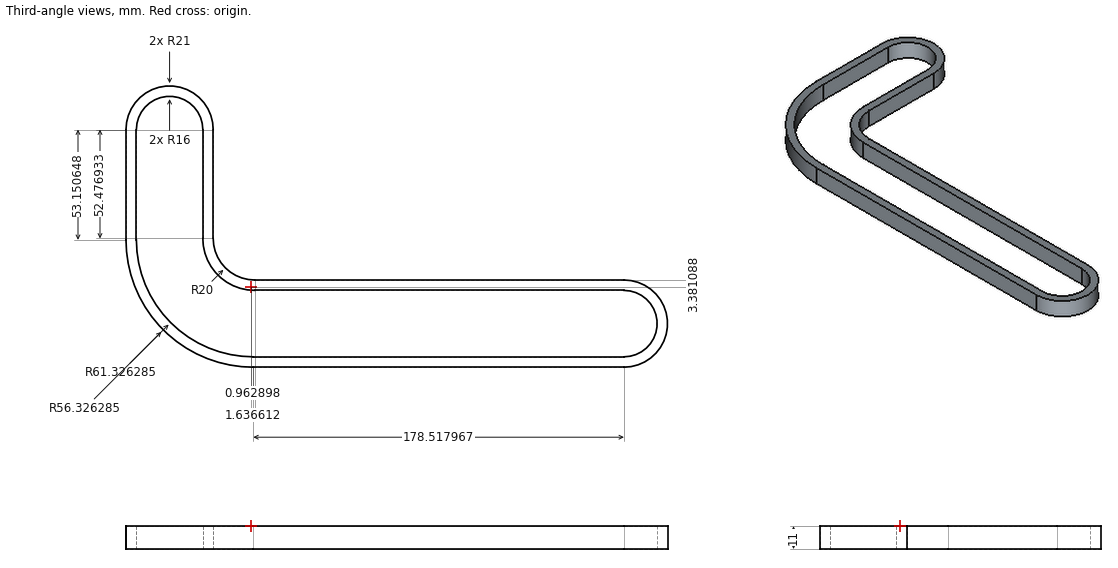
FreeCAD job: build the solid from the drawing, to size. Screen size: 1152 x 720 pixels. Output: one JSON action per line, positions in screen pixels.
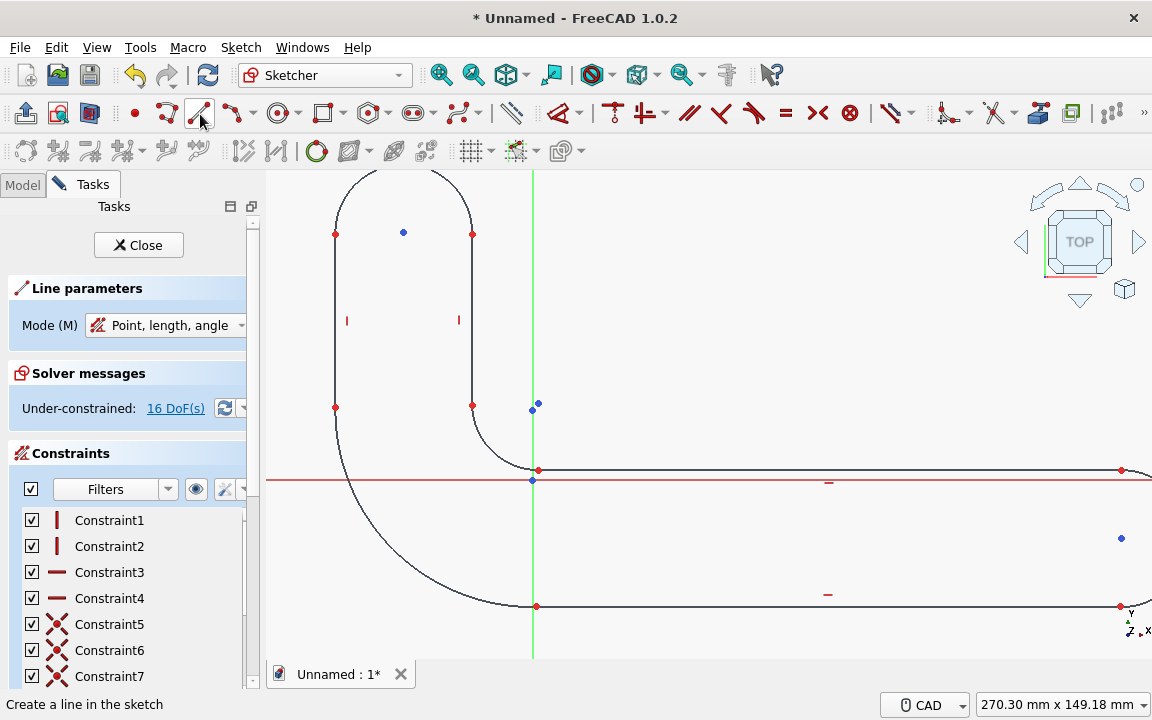
{"action": "left_click", "coordinate": [351, 406]}
{"action": "left_click", "coordinate": [351, 232]}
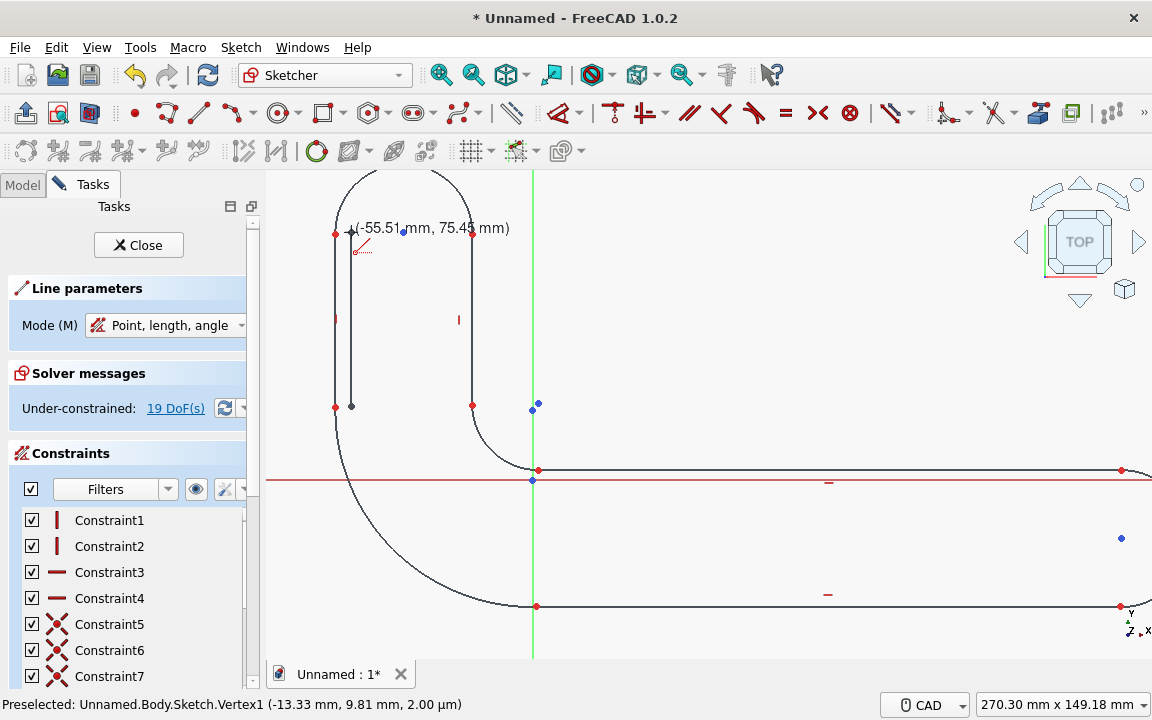
{"action": "left_click", "coordinate": [456, 232]}
{"action": "left_click", "coordinate": [456, 404]}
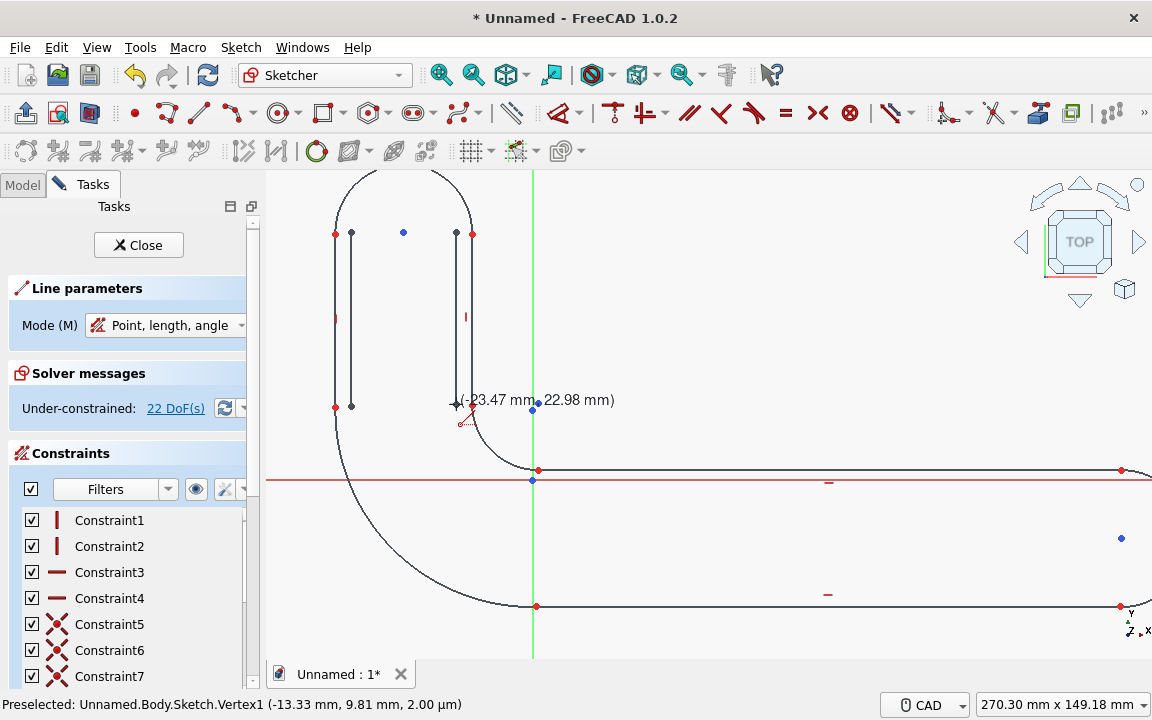
{"action": "scroll", "coordinate": [538, 486], "scroll_direction": "up", "scroll_amount": 6}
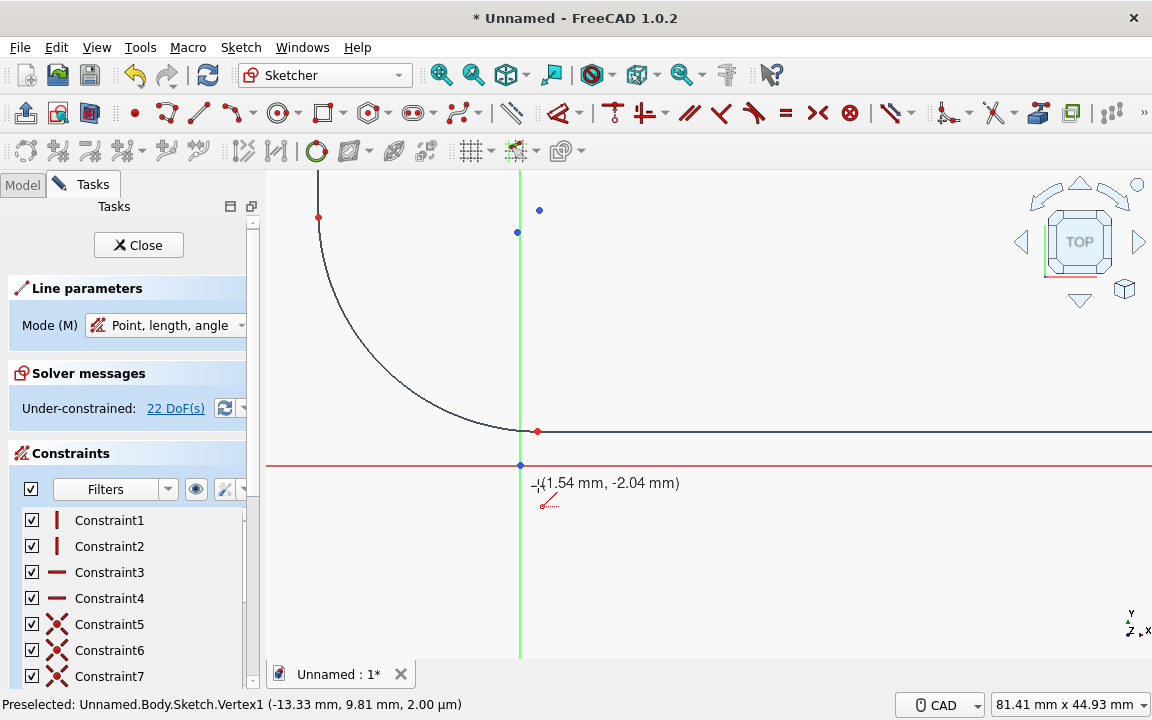
{"action": "left_click", "coordinate": [538, 483]}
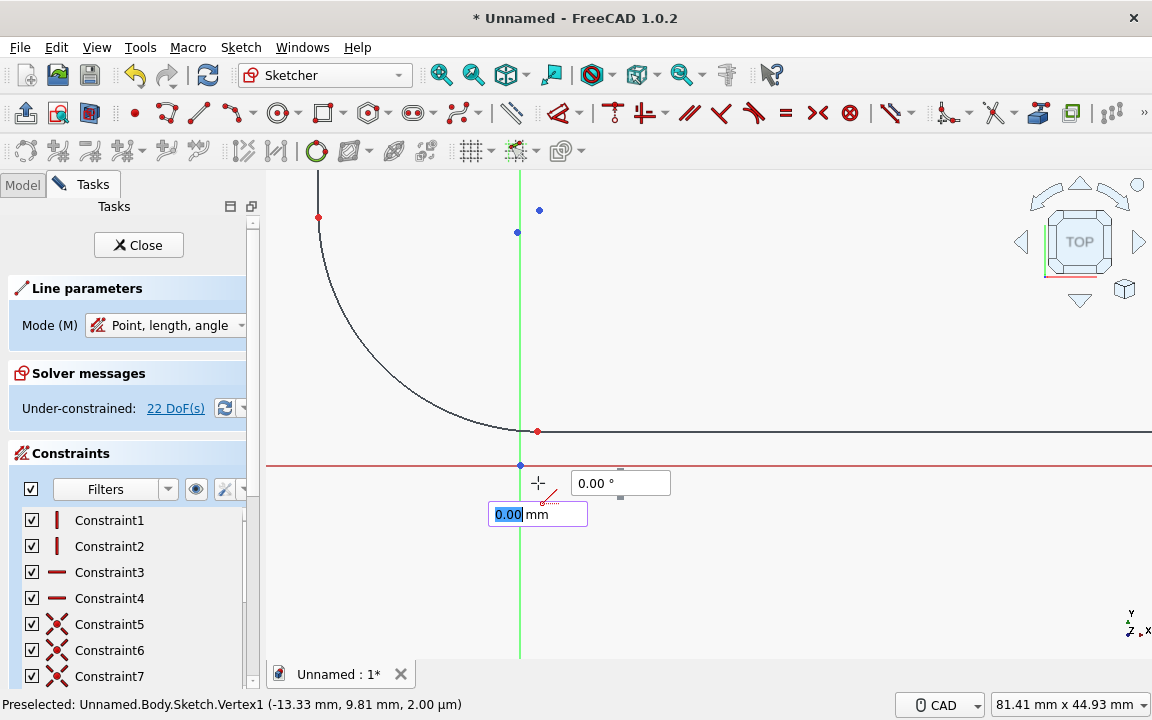
{"action": "scroll", "coordinate": [513, 467], "scroll_direction": "down", "scroll_amount": 9}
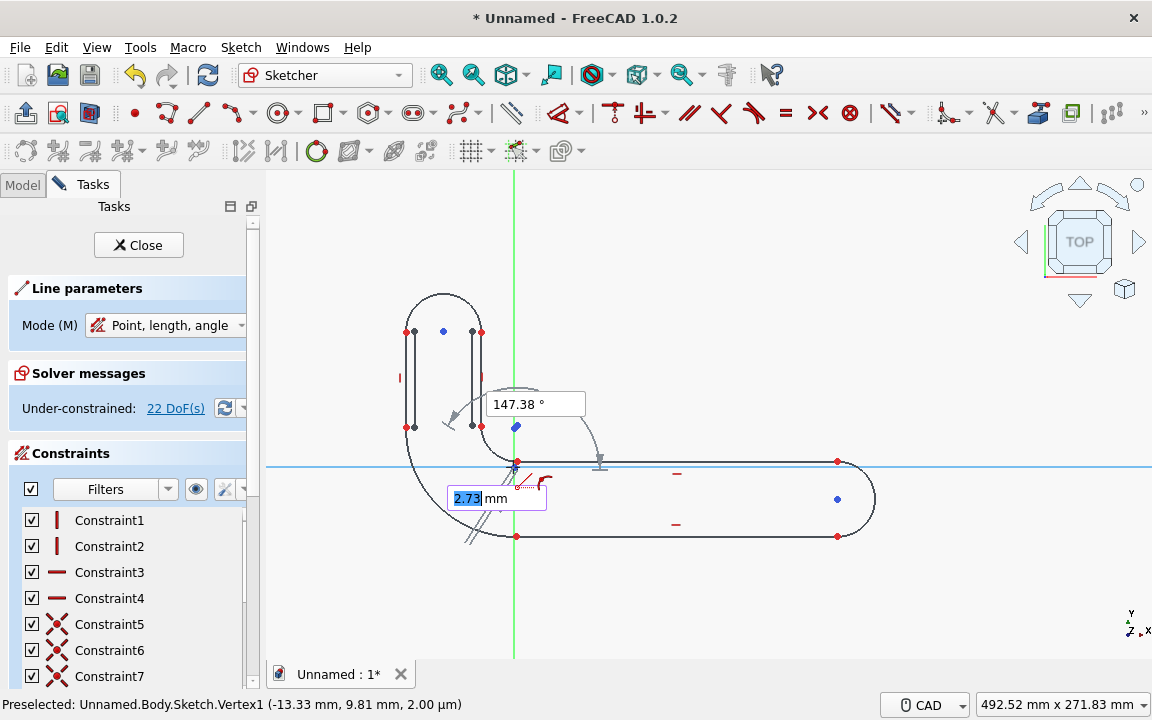
{"action": "scroll", "coordinate": [837, 470], "scroll_direction": "up", "scroll_amount": 9}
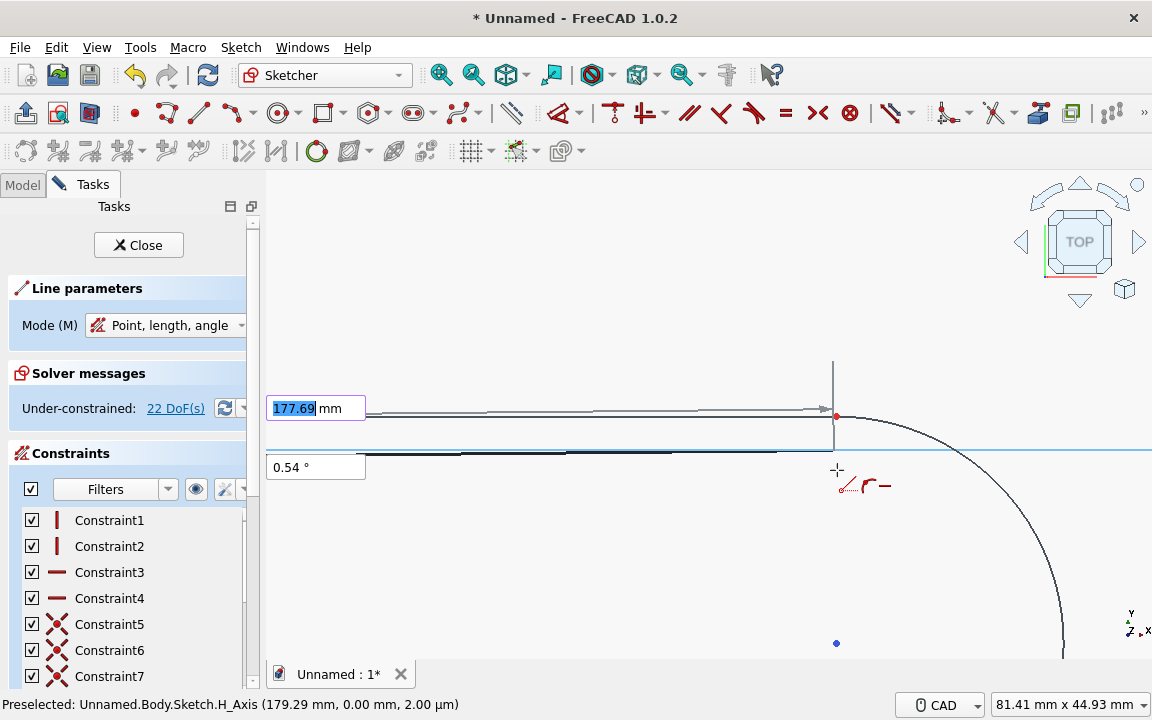
{"action": "left_click", "coordinate": [836, 468]}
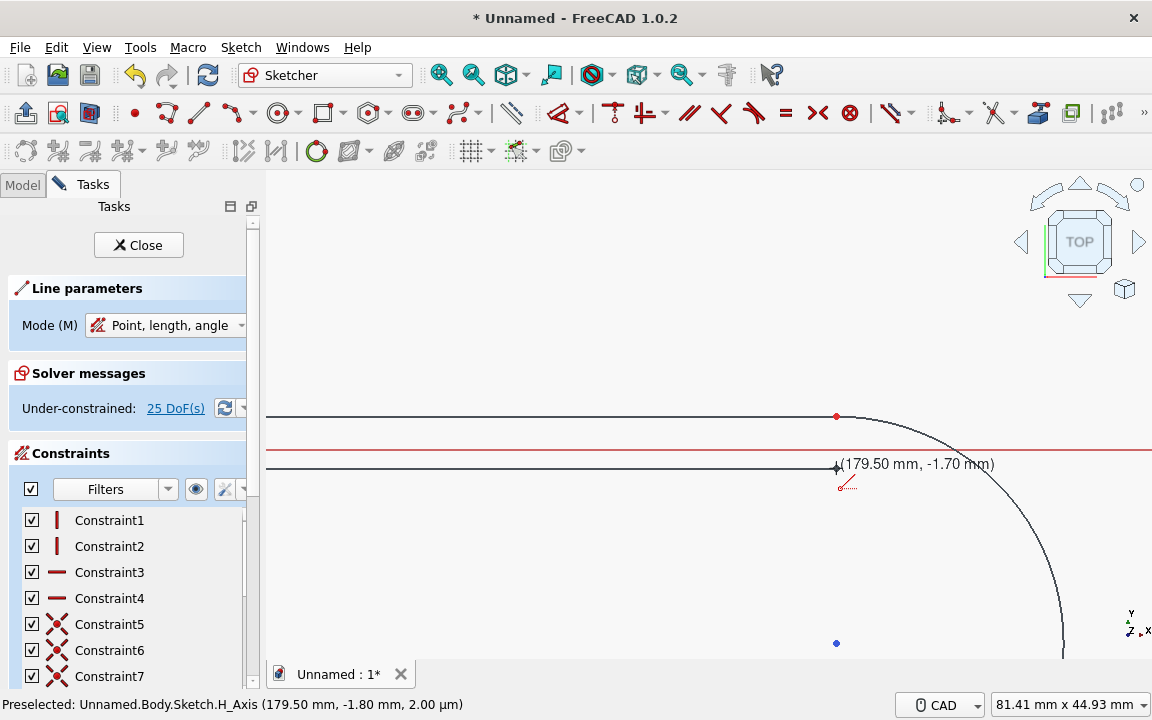
{"action": "scroll", "coordinate": [838, 470], "scroll_direction": "down", "scroll_amount": 9}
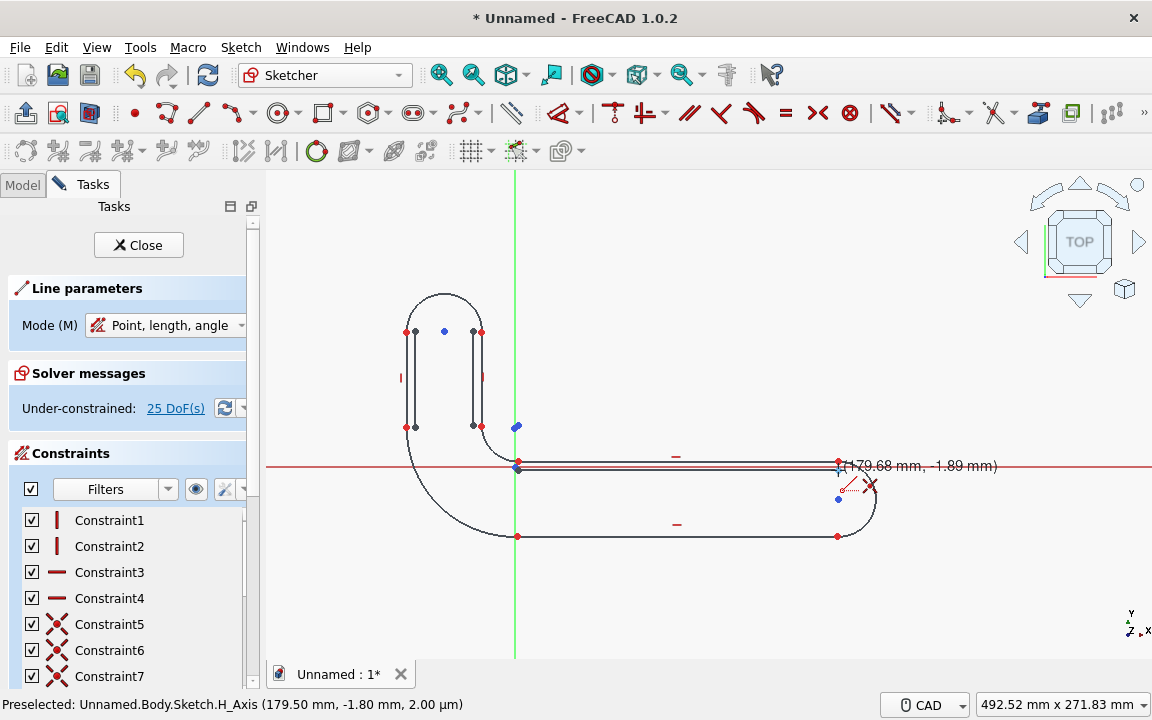
{"action": "scroll", "coordinate": [838, 528], "scroll_direction": "up", "scroll_amount": 3}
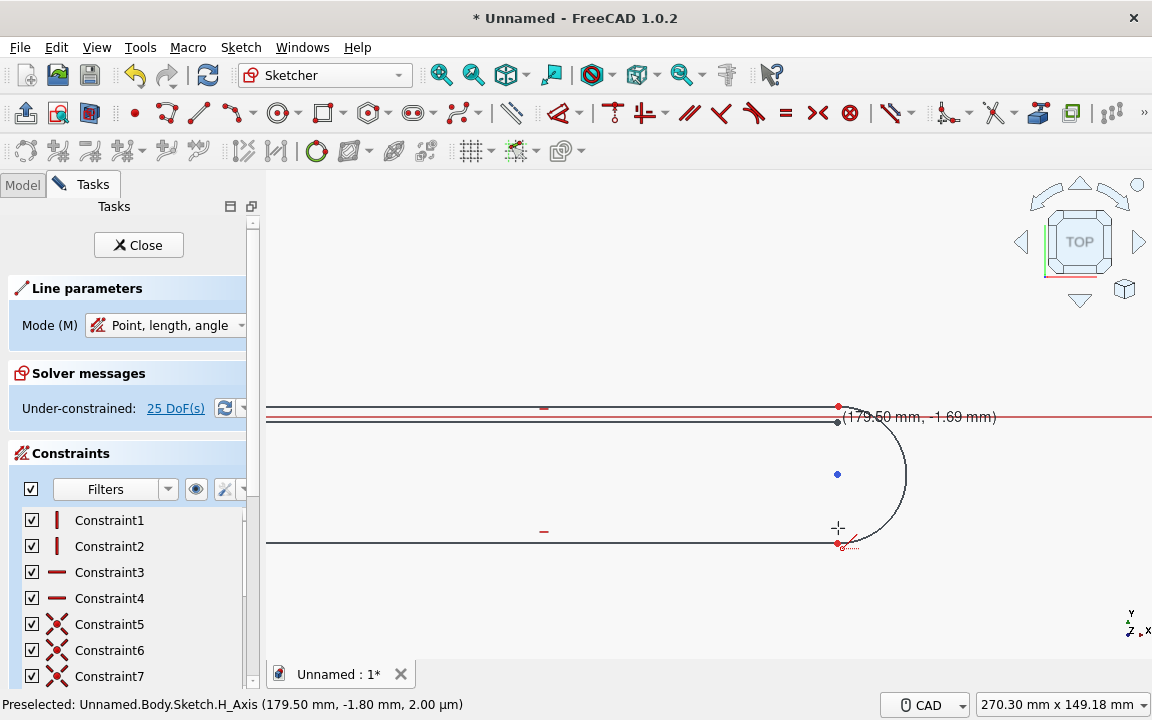
{"action": "left_click", "coordinate": [838, 527]}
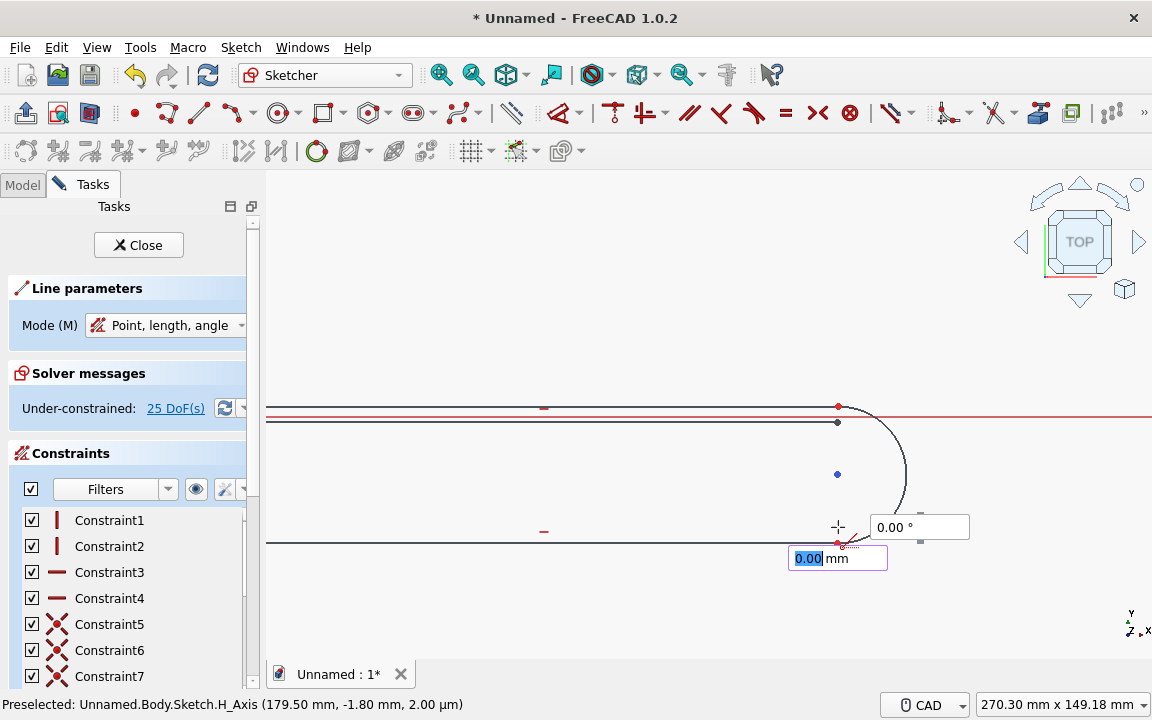
{"action": "scroll", "coordinate": [837, 528], "scroll_direction": "down", "scroll_amount": 3}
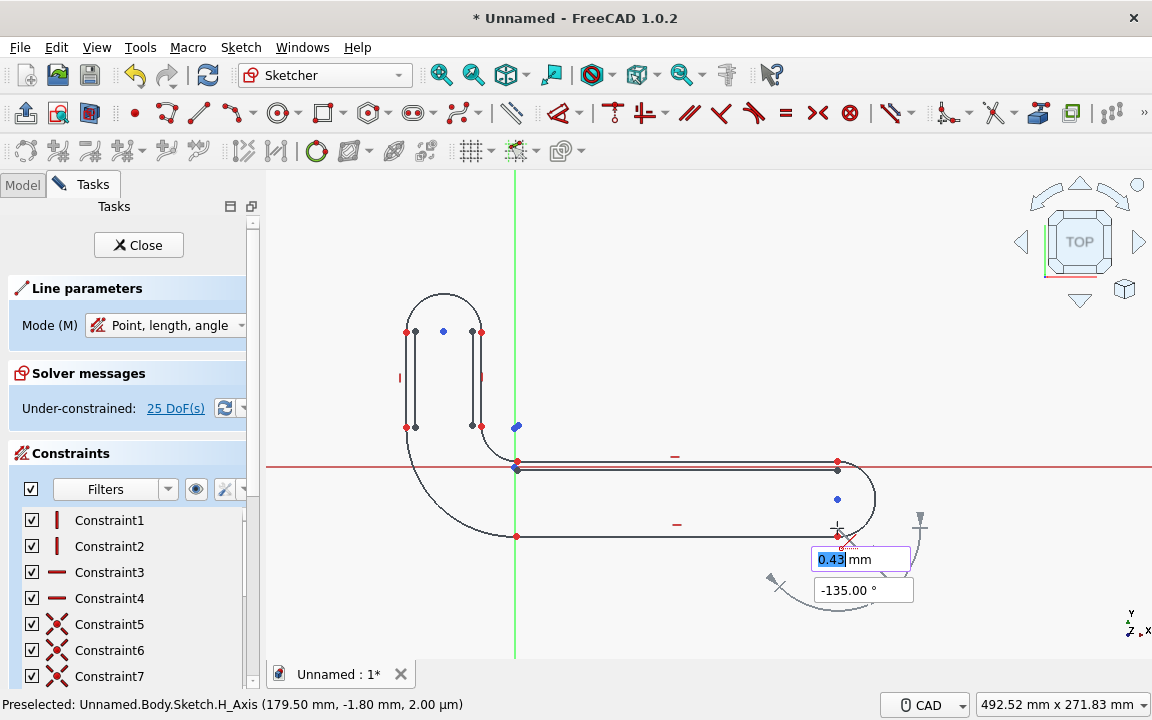
{"action": "scroll", "coordinate": [517, 528], "scroll_direction": "up", "scroll_amount": 12}